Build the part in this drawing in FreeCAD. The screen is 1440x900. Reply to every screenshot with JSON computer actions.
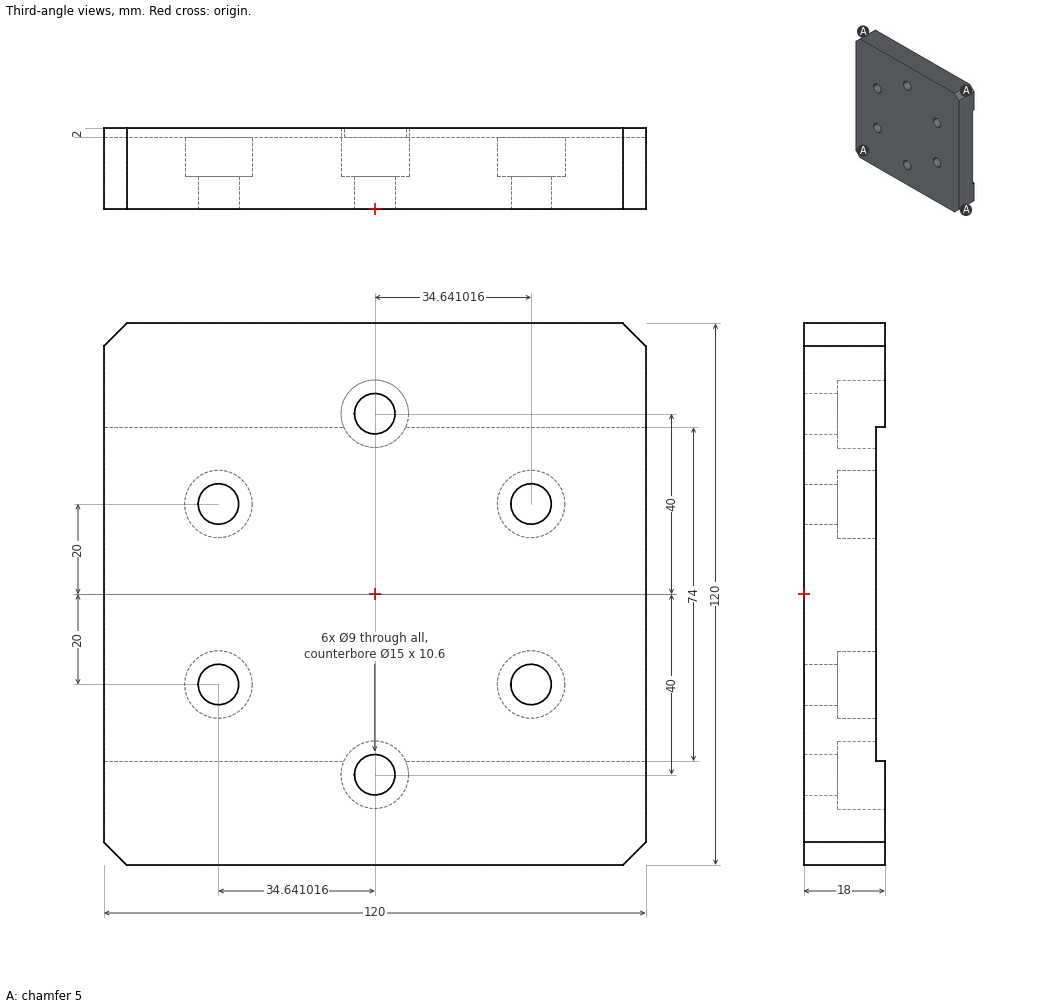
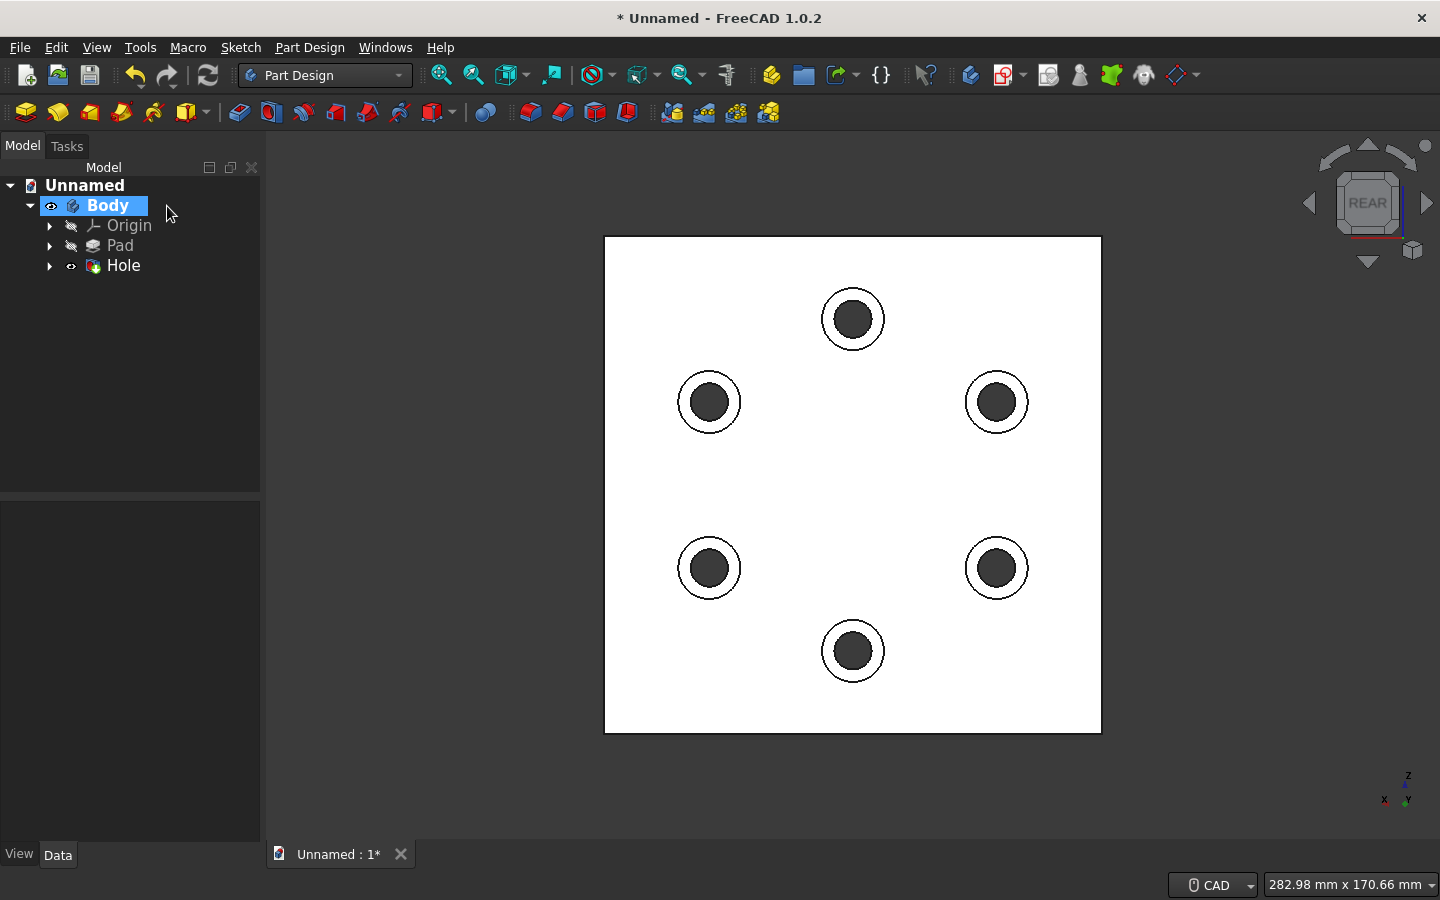
{"action": "left_click", "coordinate": [853, 484]}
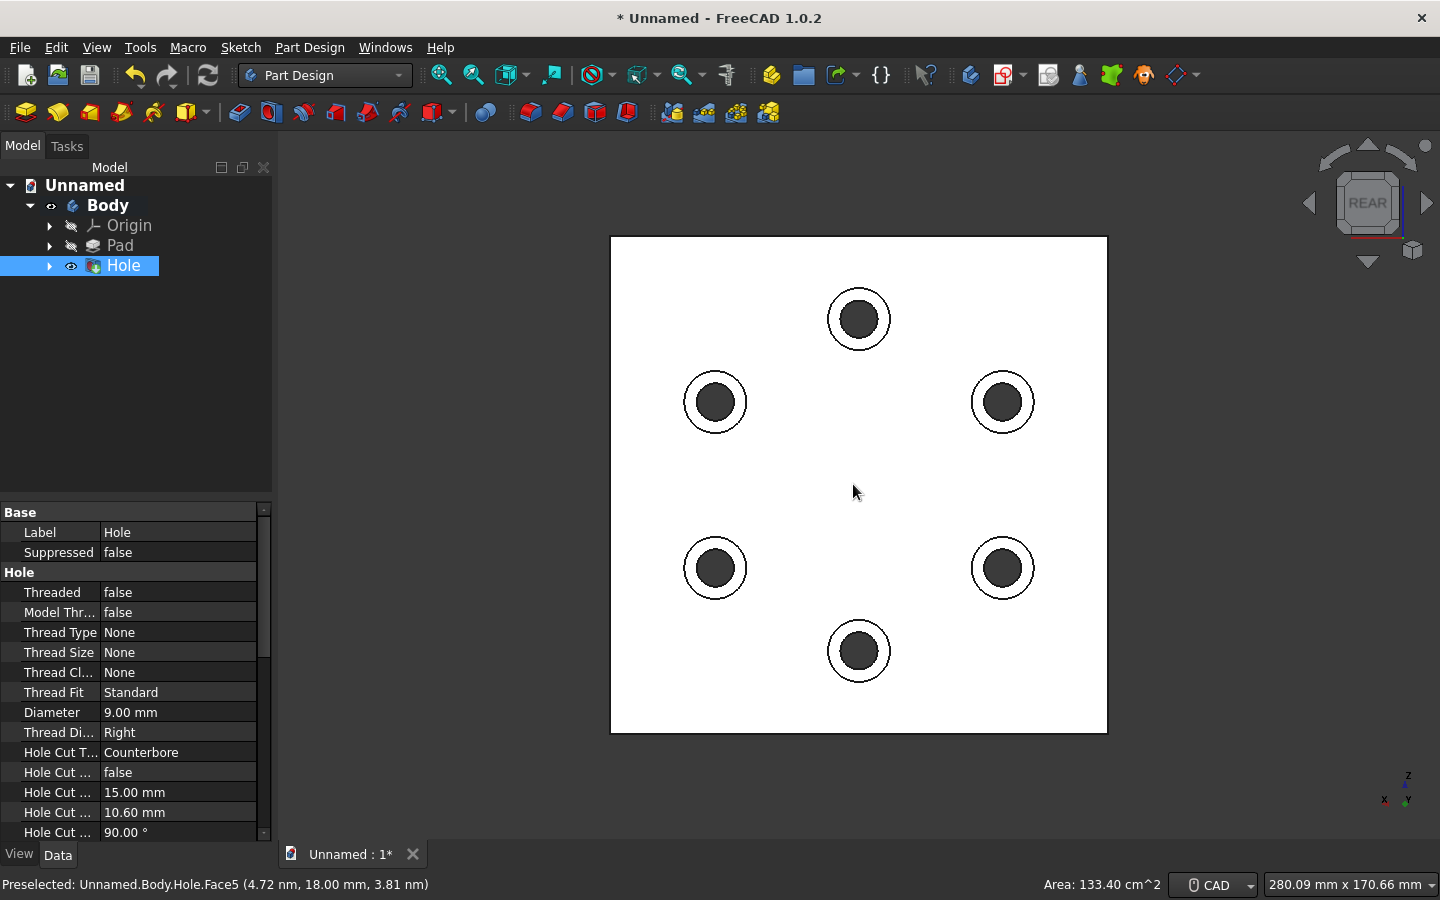
{"action": "left_click", "coordinate": [1004, 76]}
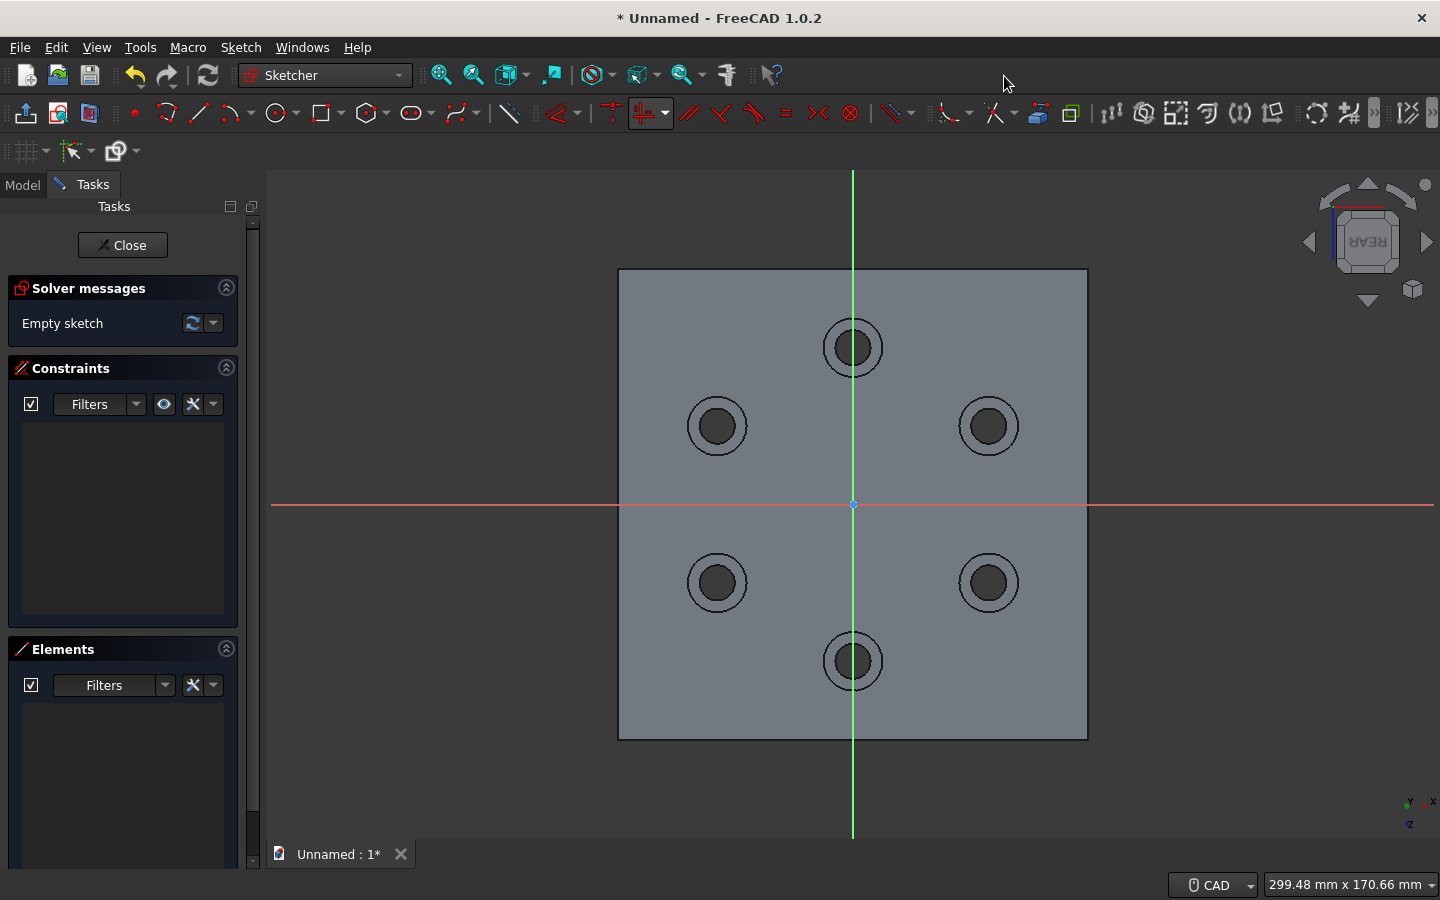
{"action": "scroll", "coordinate": [992, 504], "scroll_direction": "up", "scroll_amount": 2}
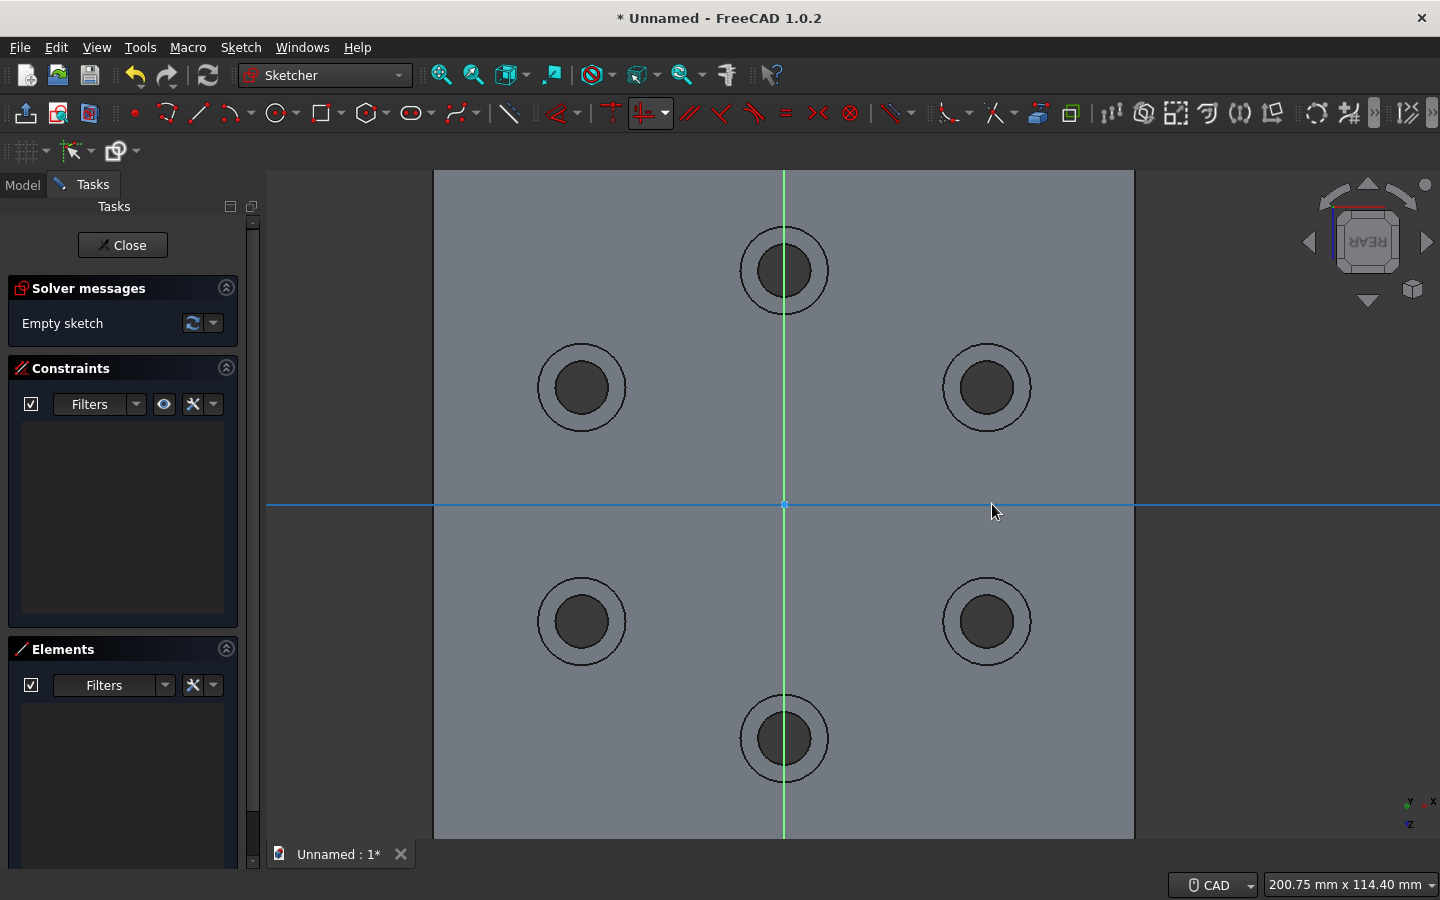
{"action": "key", "text": "g v"}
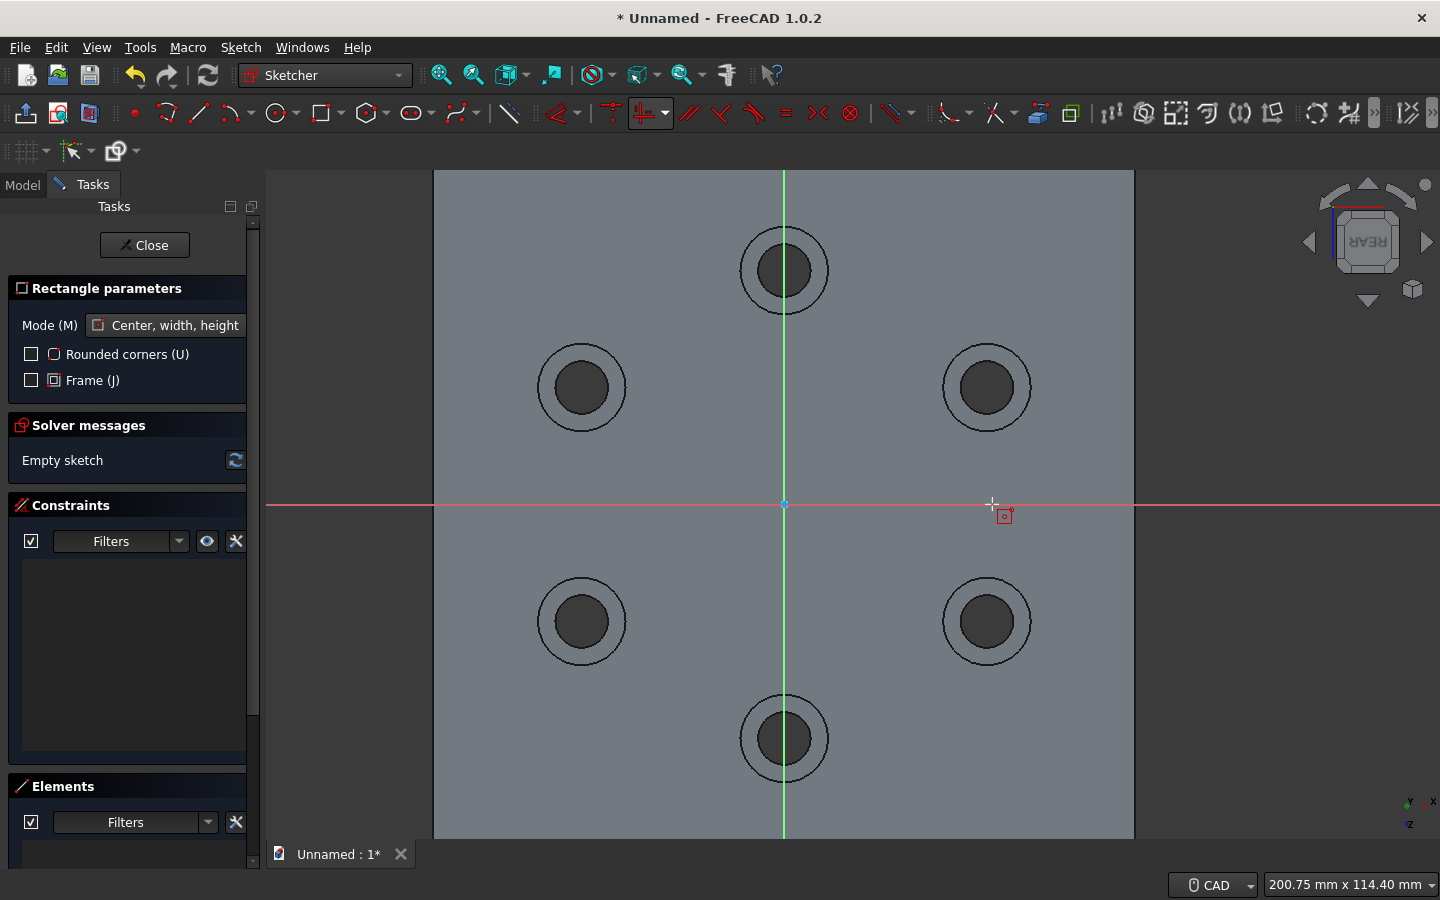
{"action": "left_click", "coordinate": [784, 504]}
{"action": "mouse_move", "coordinate": [1135, 288]}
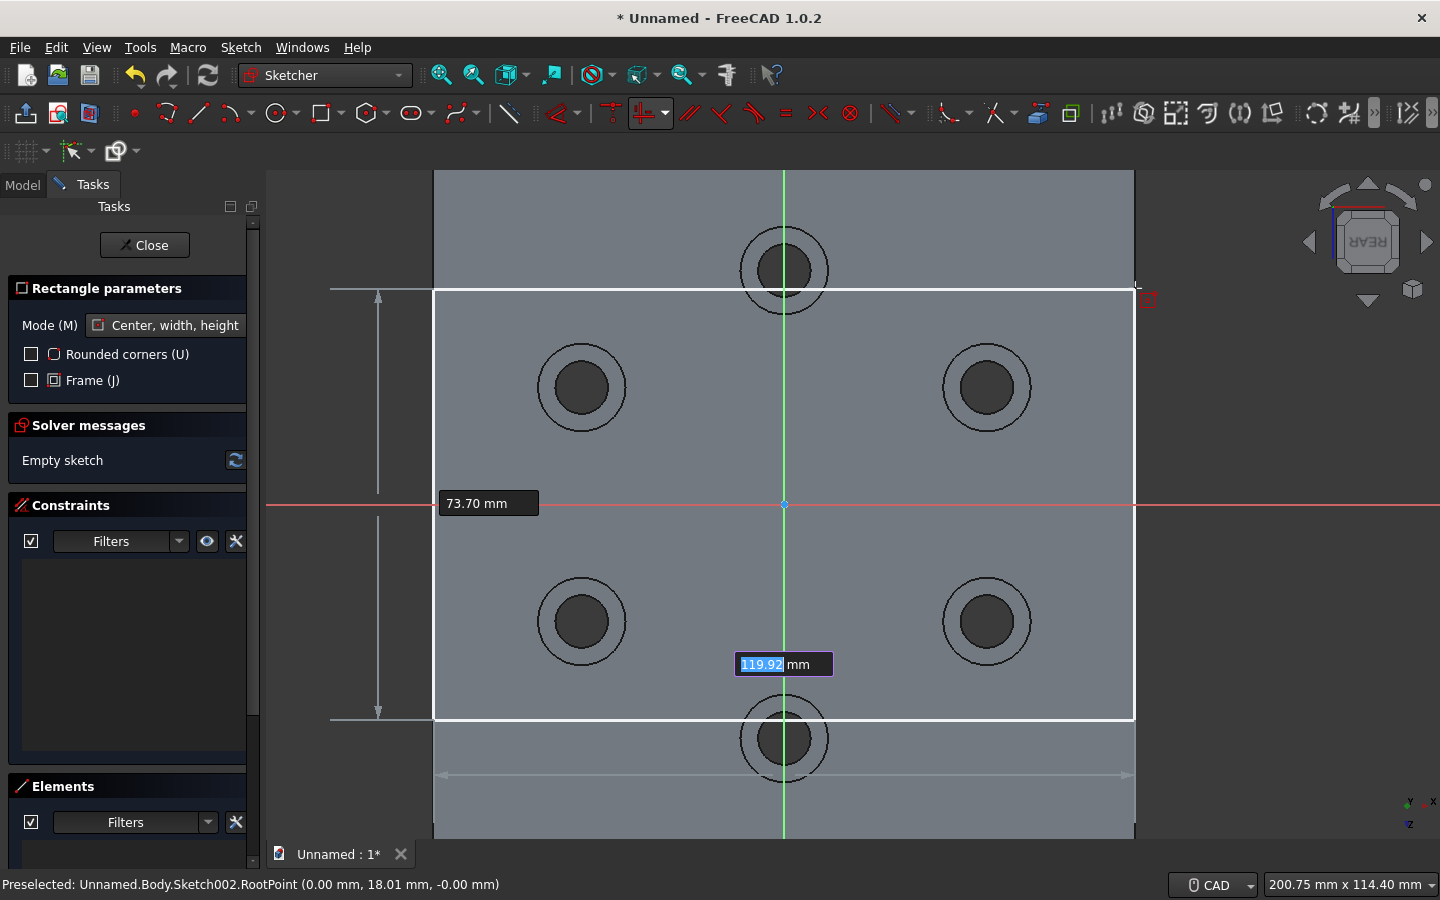
{"action": "type", "text": "120"}
{"action": "key", "text": "Tab"}
{"action": "type", "text": "74"}
{"action": "key", "text": "Return"}
{"action": "key", "text": "Escape"}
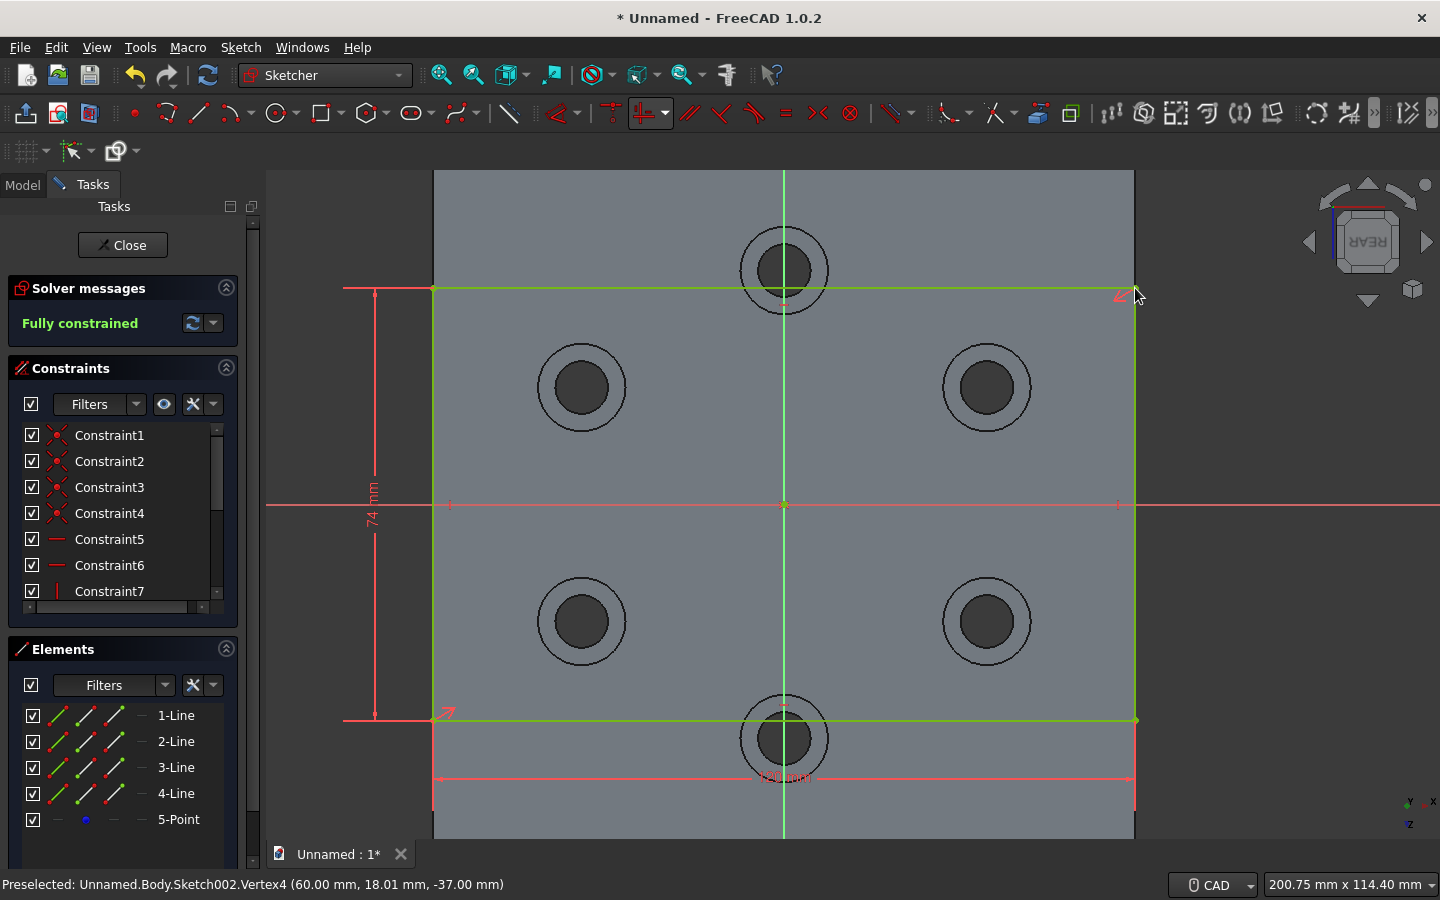
{"action": "left_click", "coordinate": [123, 245]}